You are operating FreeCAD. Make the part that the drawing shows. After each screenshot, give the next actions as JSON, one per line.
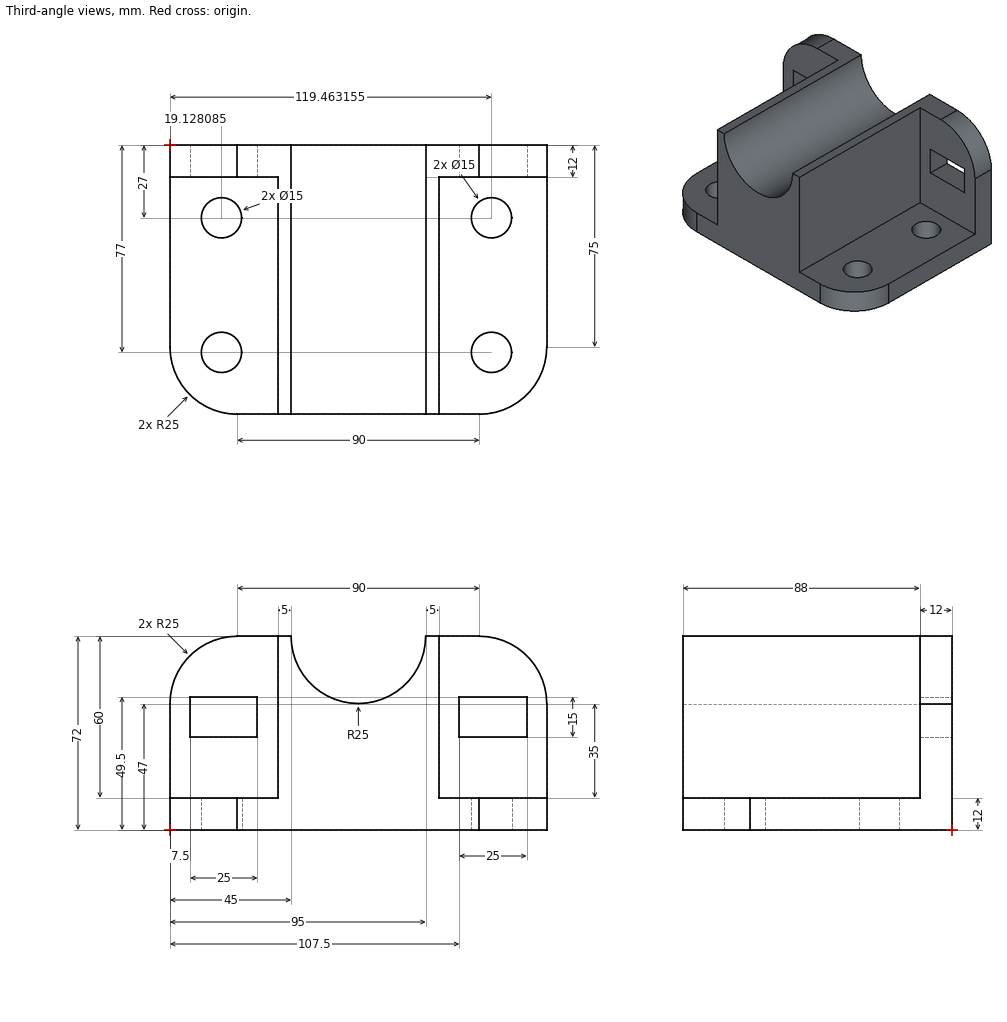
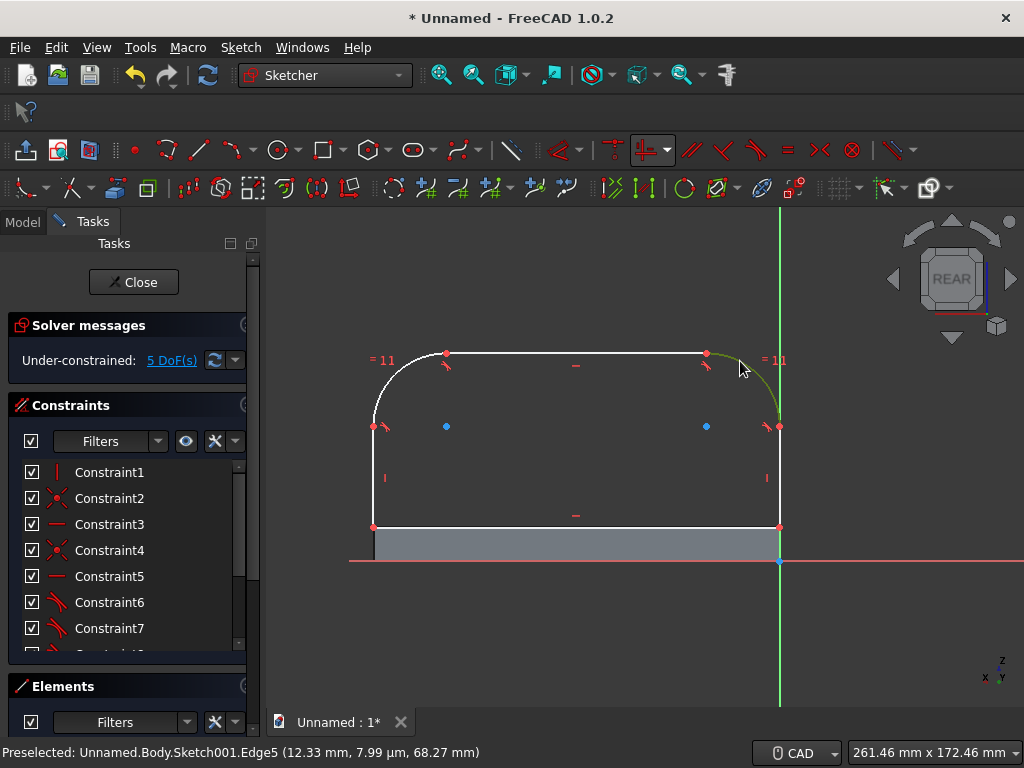
{"action": "key", "text": "k r"}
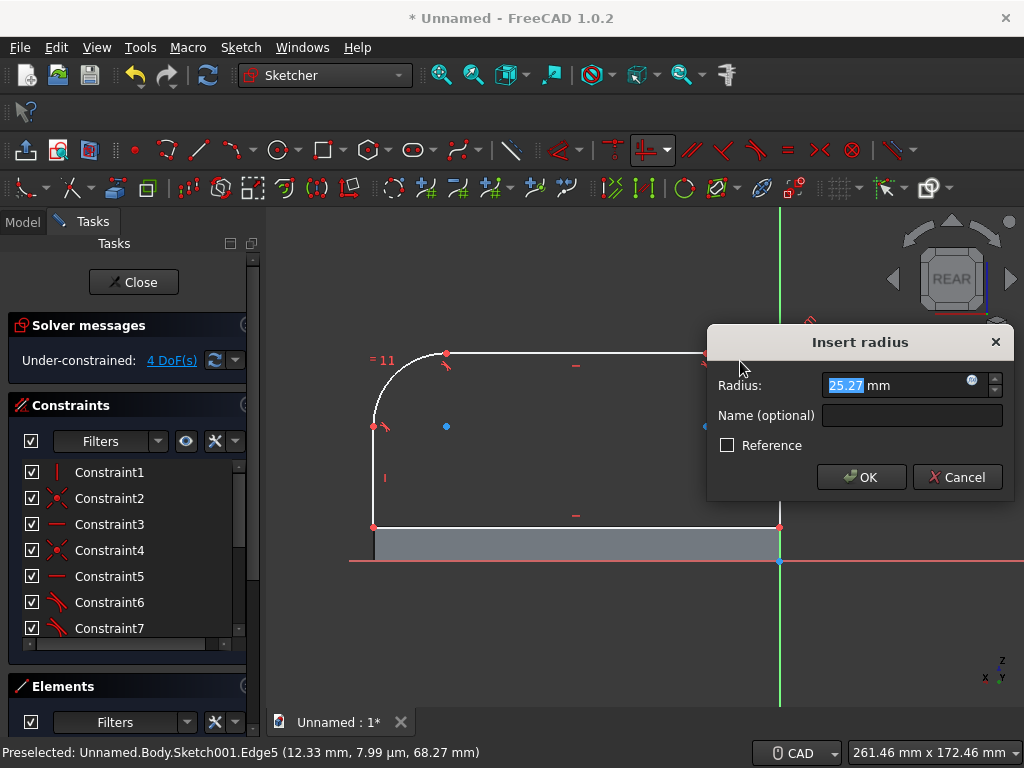
{"action": "type", "text": "25"}
{"action": "key", "text": "Return"}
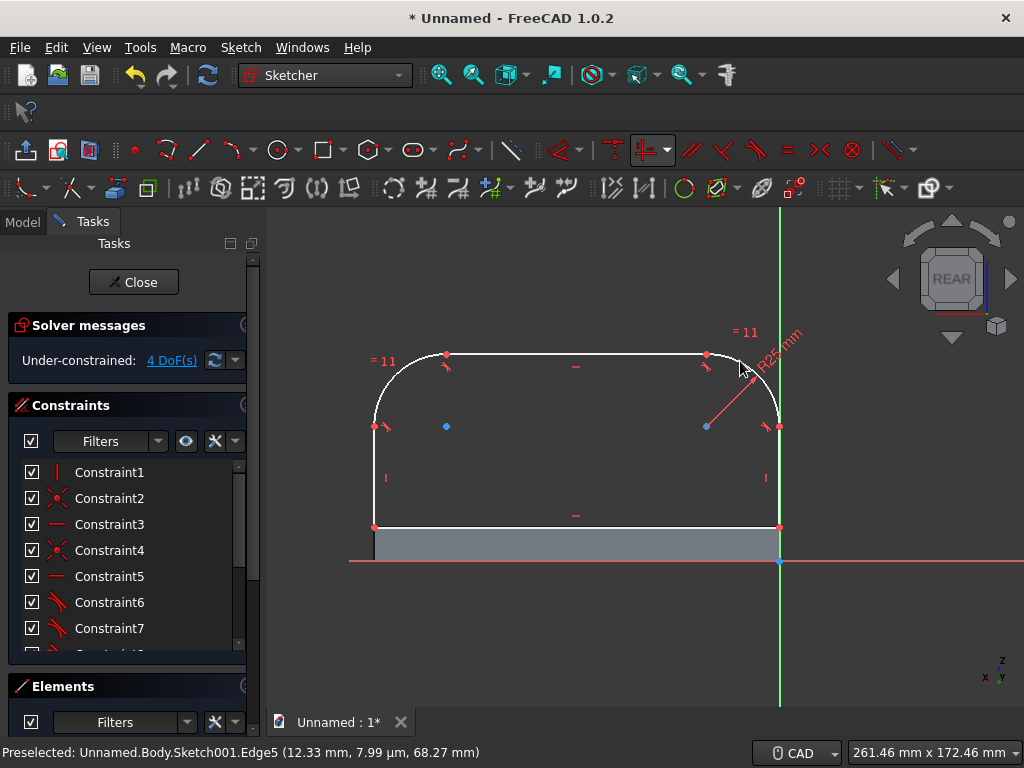
{"action": "left_click", "coordinate": [779, 528]}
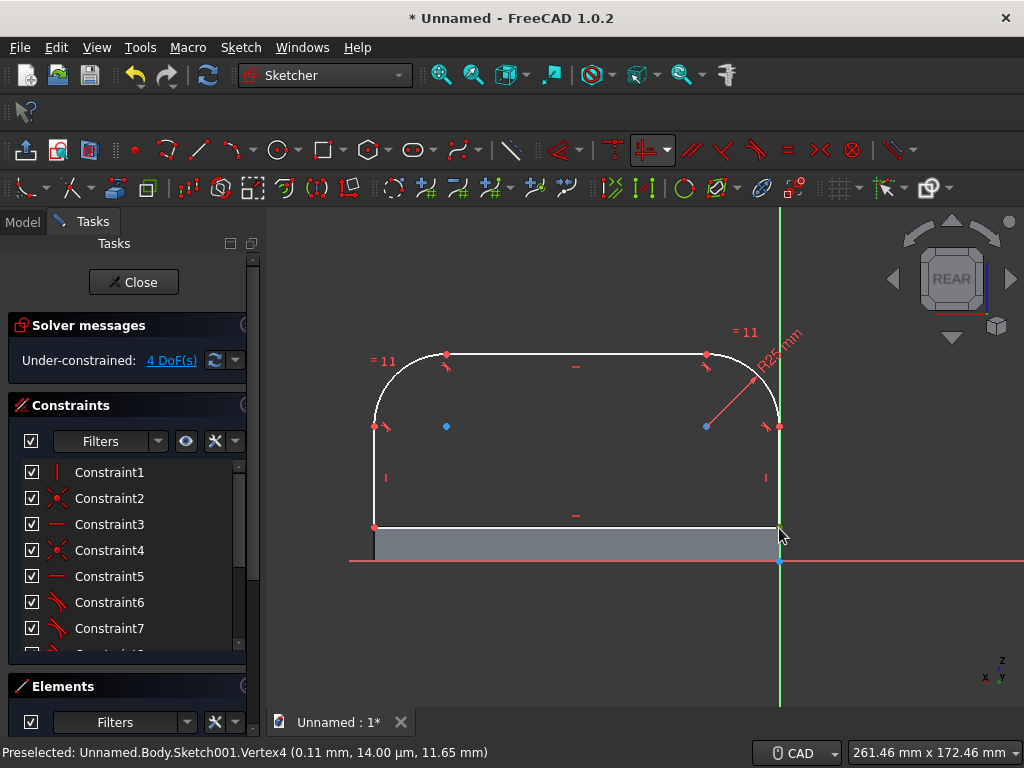
{"action": "left_click", "coordinate": [780, 647]}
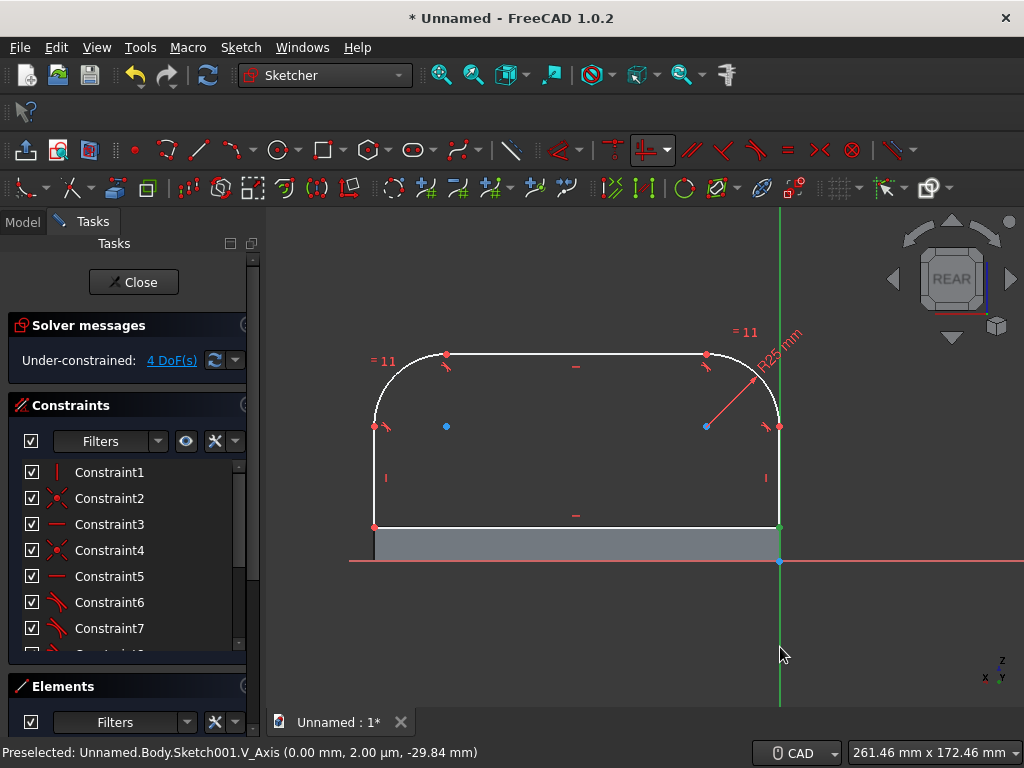
{"action": "key", "text": "c"}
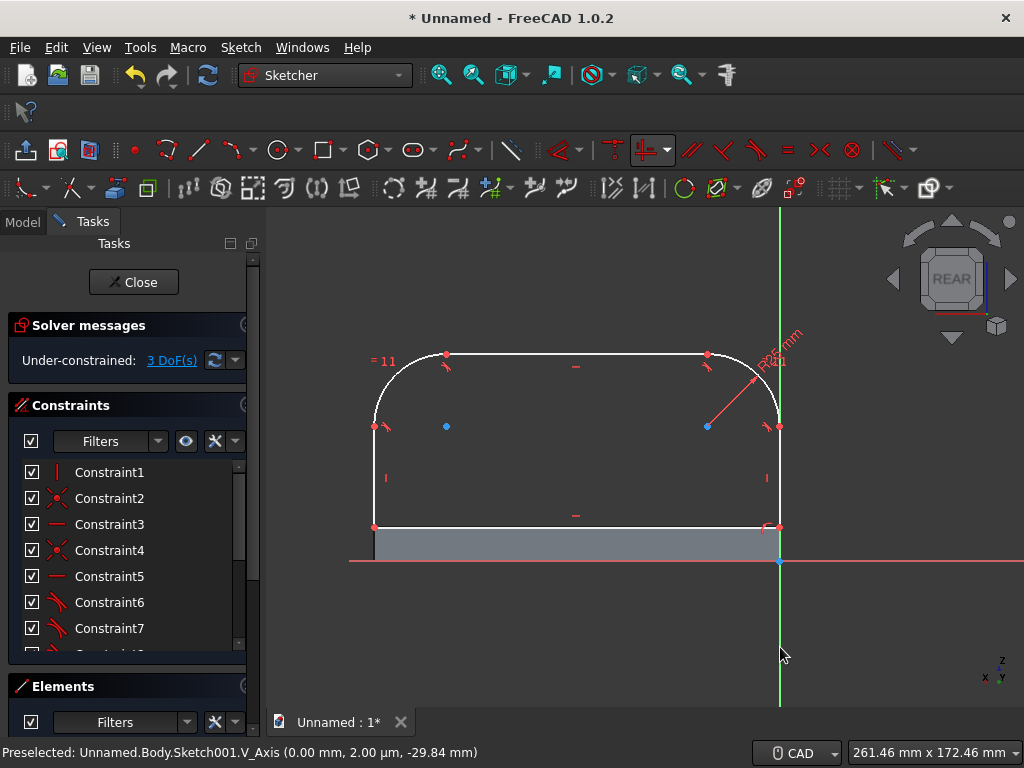
{"action": "left_click", "coordinate": [374, 457]}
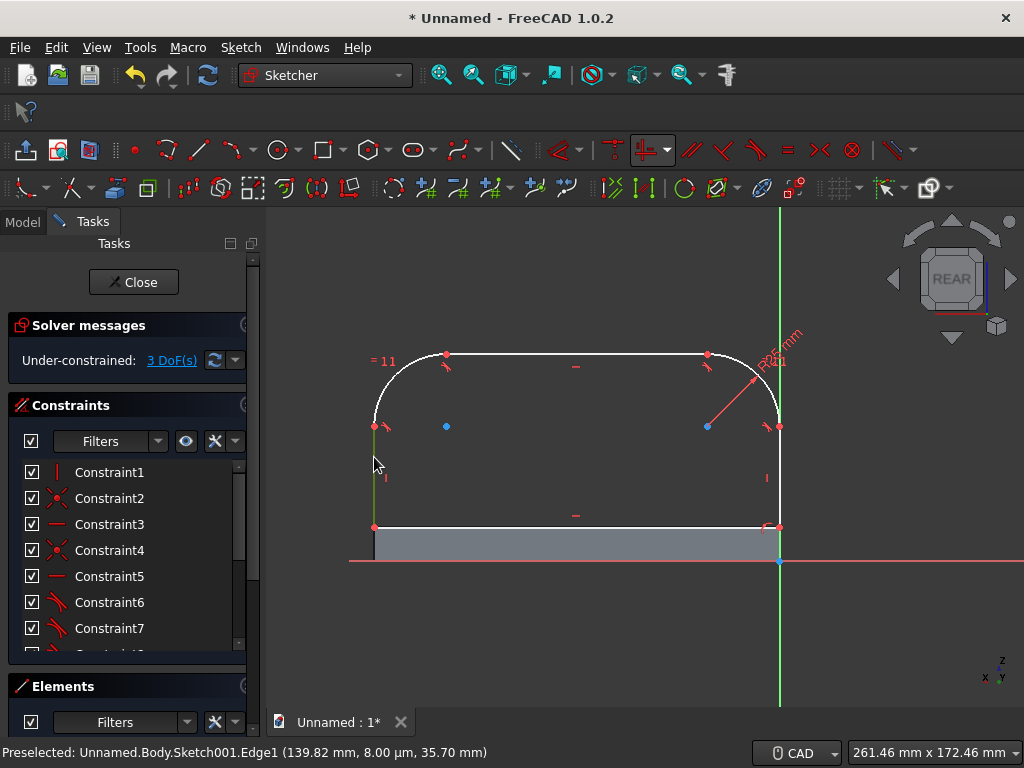
{"action": "left_click", "coordinate": [582, 150]}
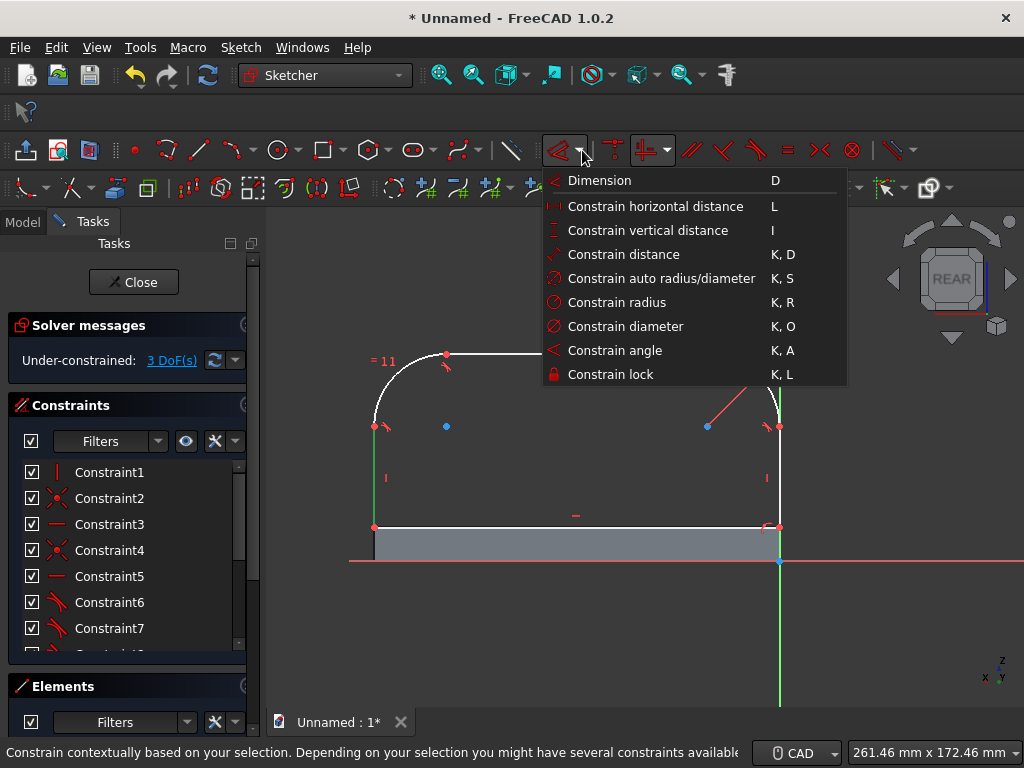
{"action": "left_click", "coordinate": [695, 230]}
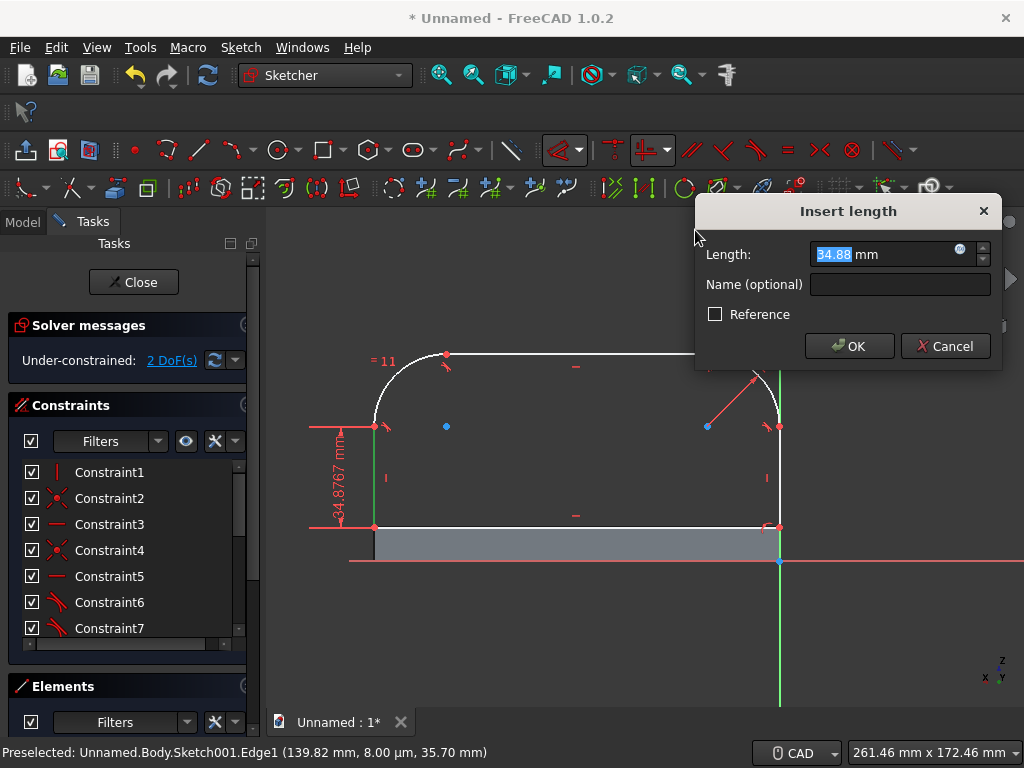
{"action": "type", "text": "35"}
{"action": "key", "text": "Return"}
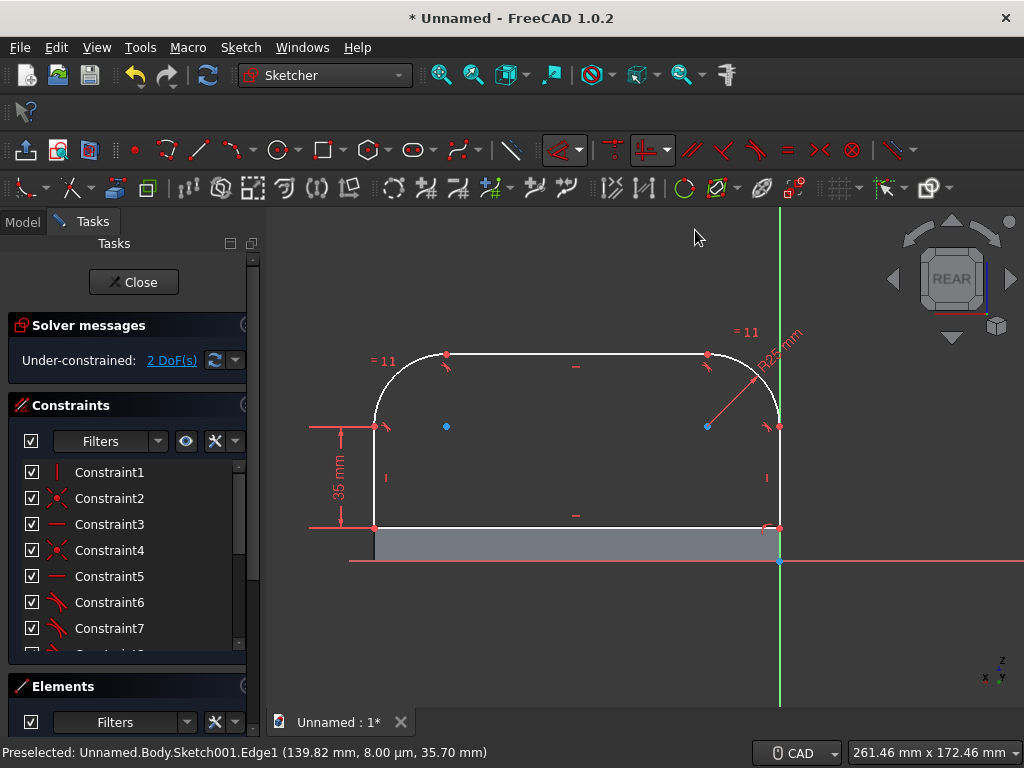
{"action": "left_click", "coordinate": [629, 354]}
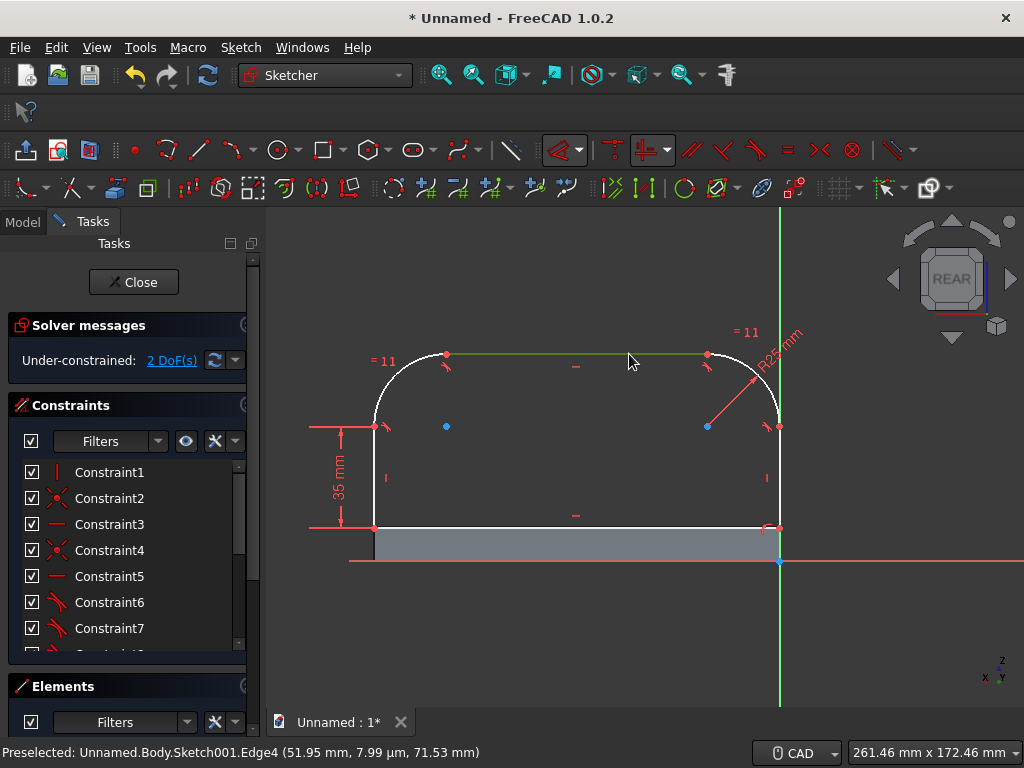
{"action": "key", "text": "l"}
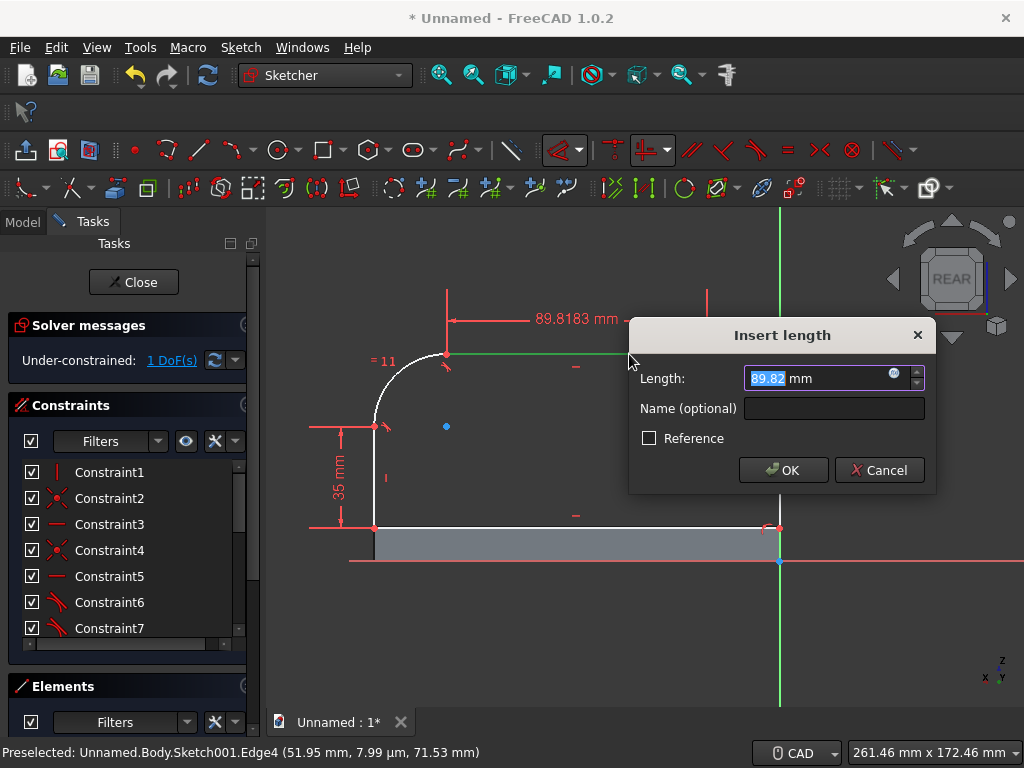
{"action": "type", "text": "90"}
{"action": "key", "text": "Return"}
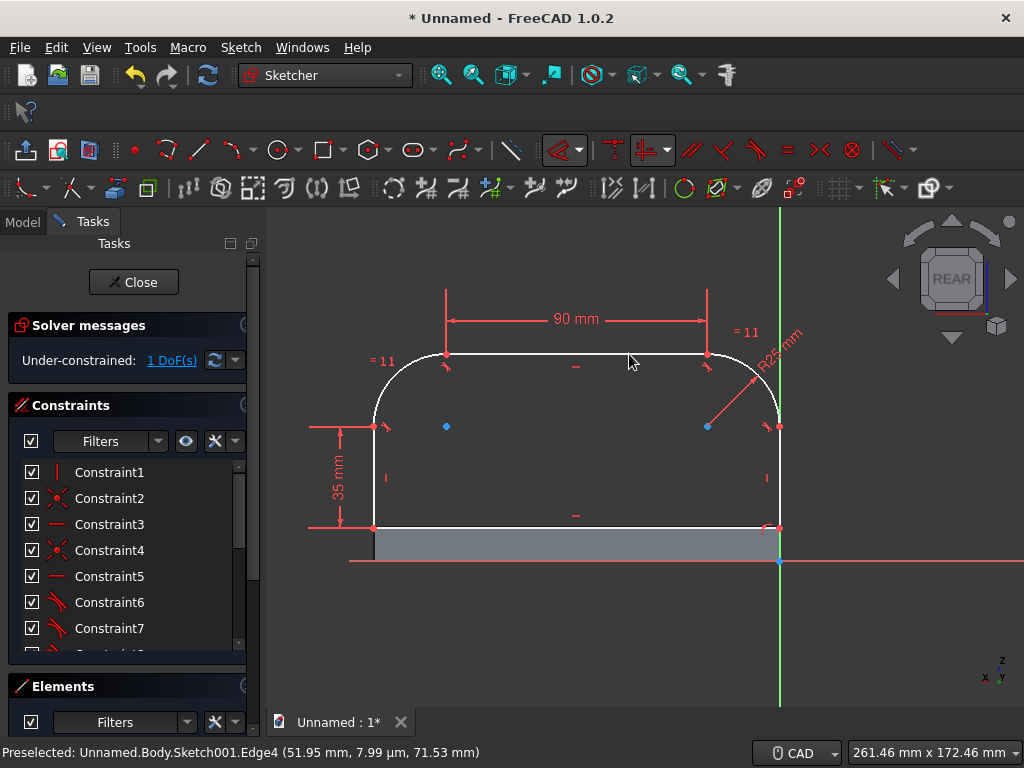
{"action": "left_click", "coordinate": [374, 427]}